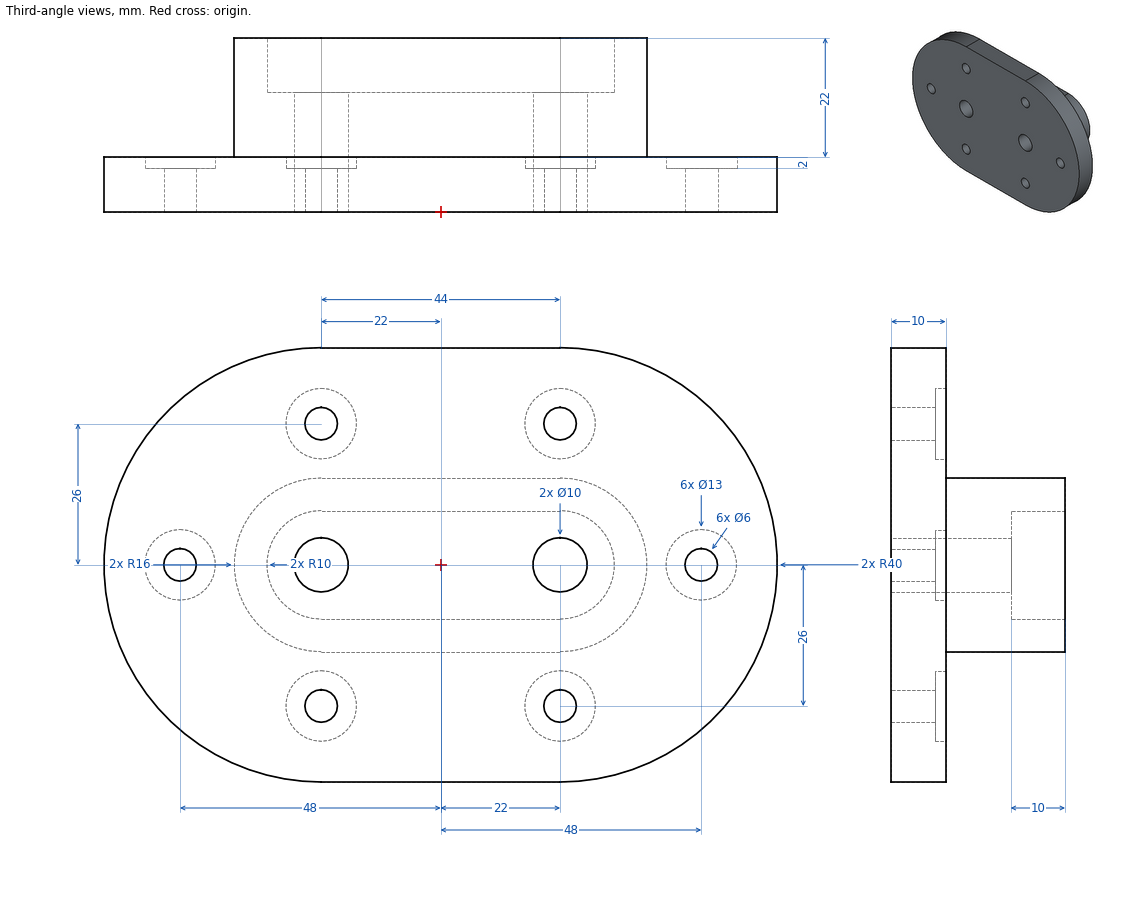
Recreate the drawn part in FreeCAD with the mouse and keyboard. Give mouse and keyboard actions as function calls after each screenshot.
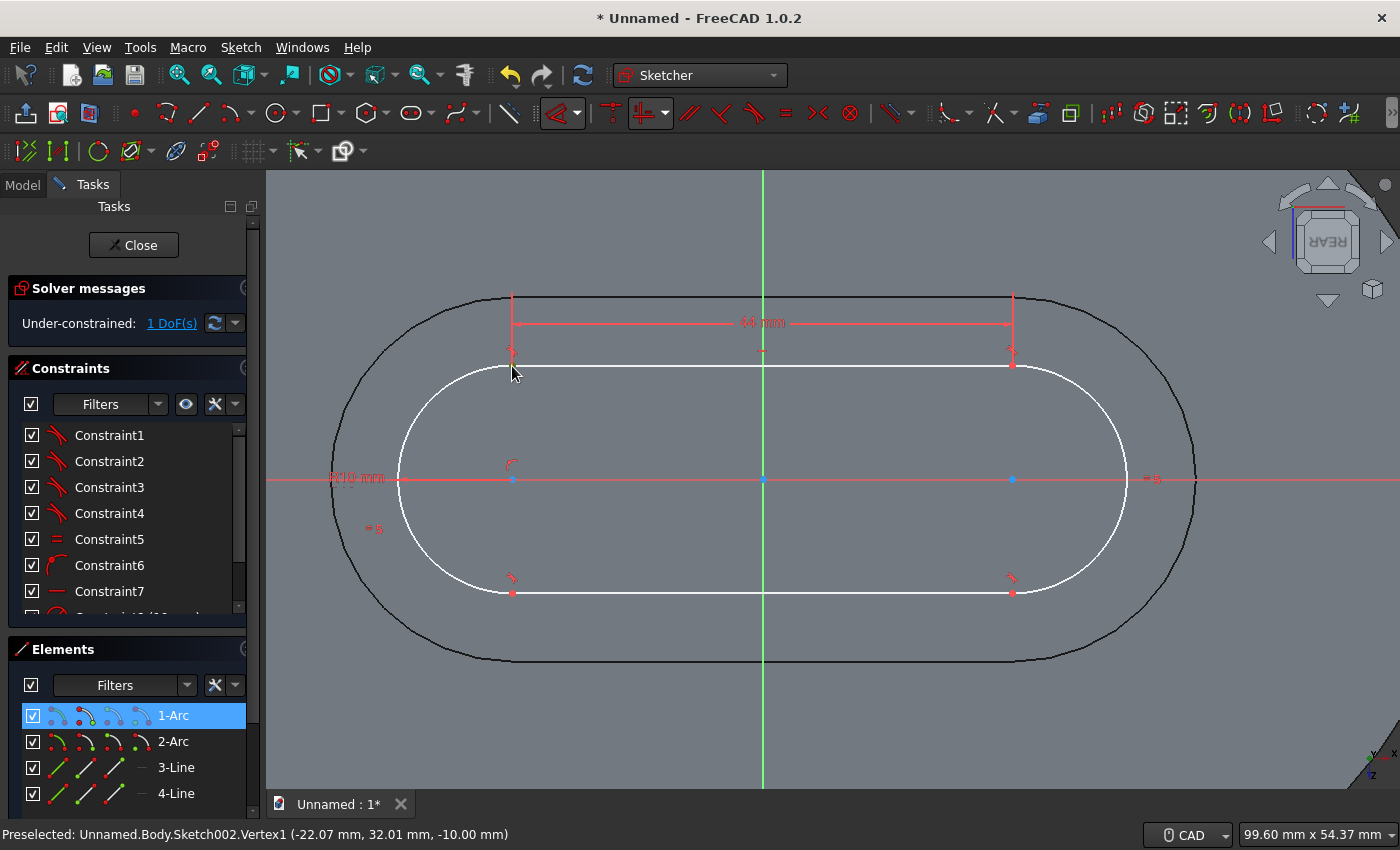
key(l)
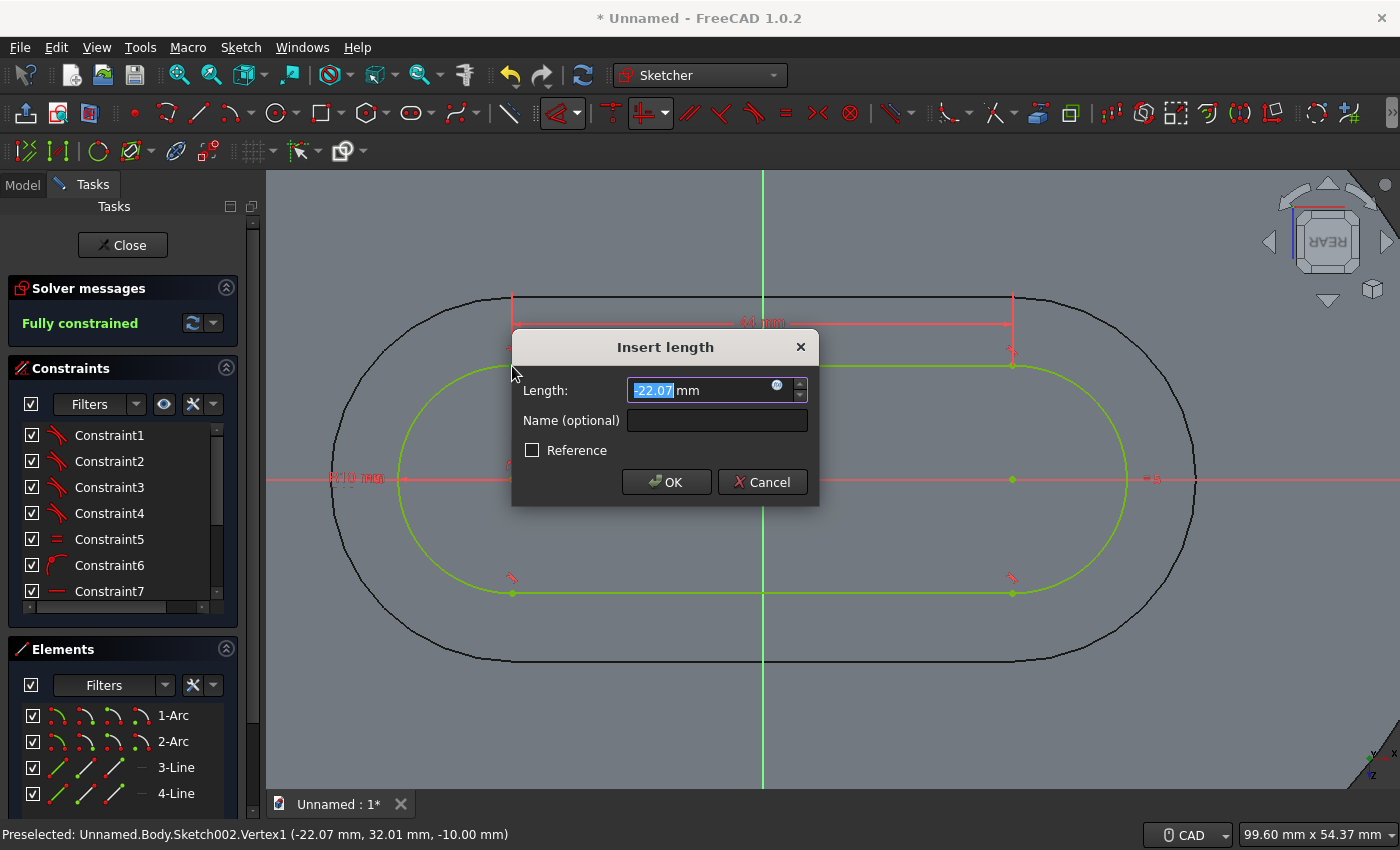
text(-22)
key(Return)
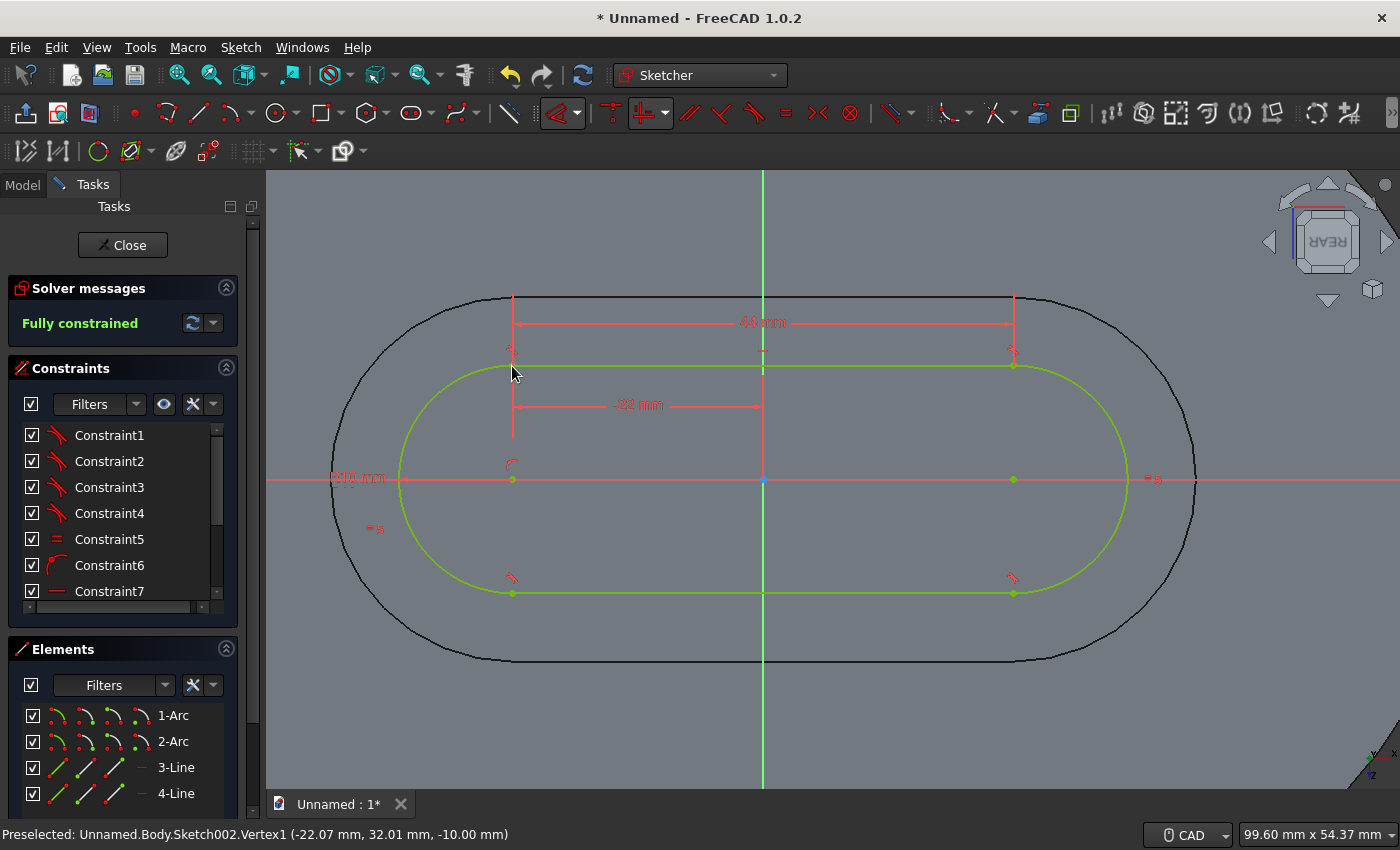
click(123, 245)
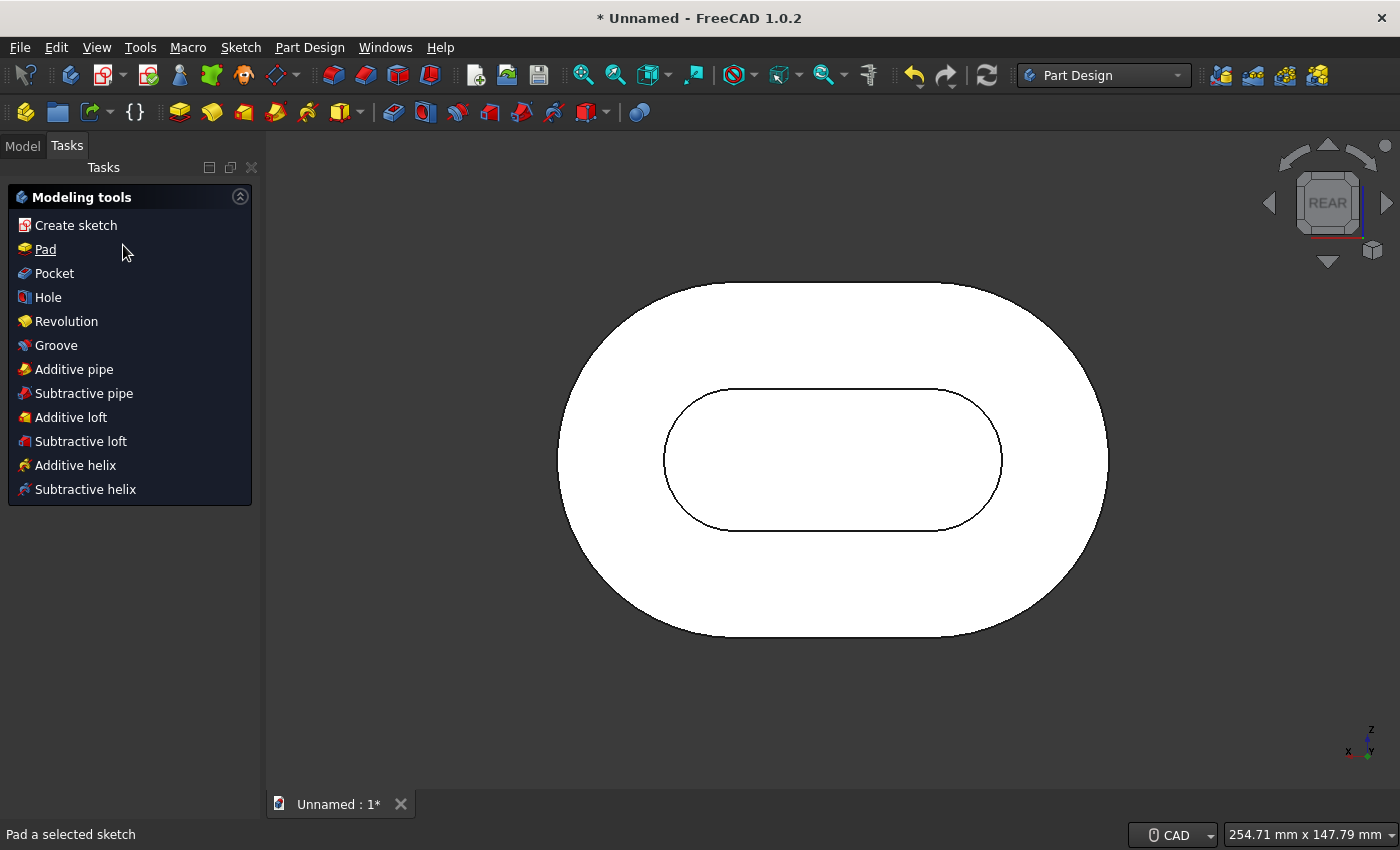
click(394, 112)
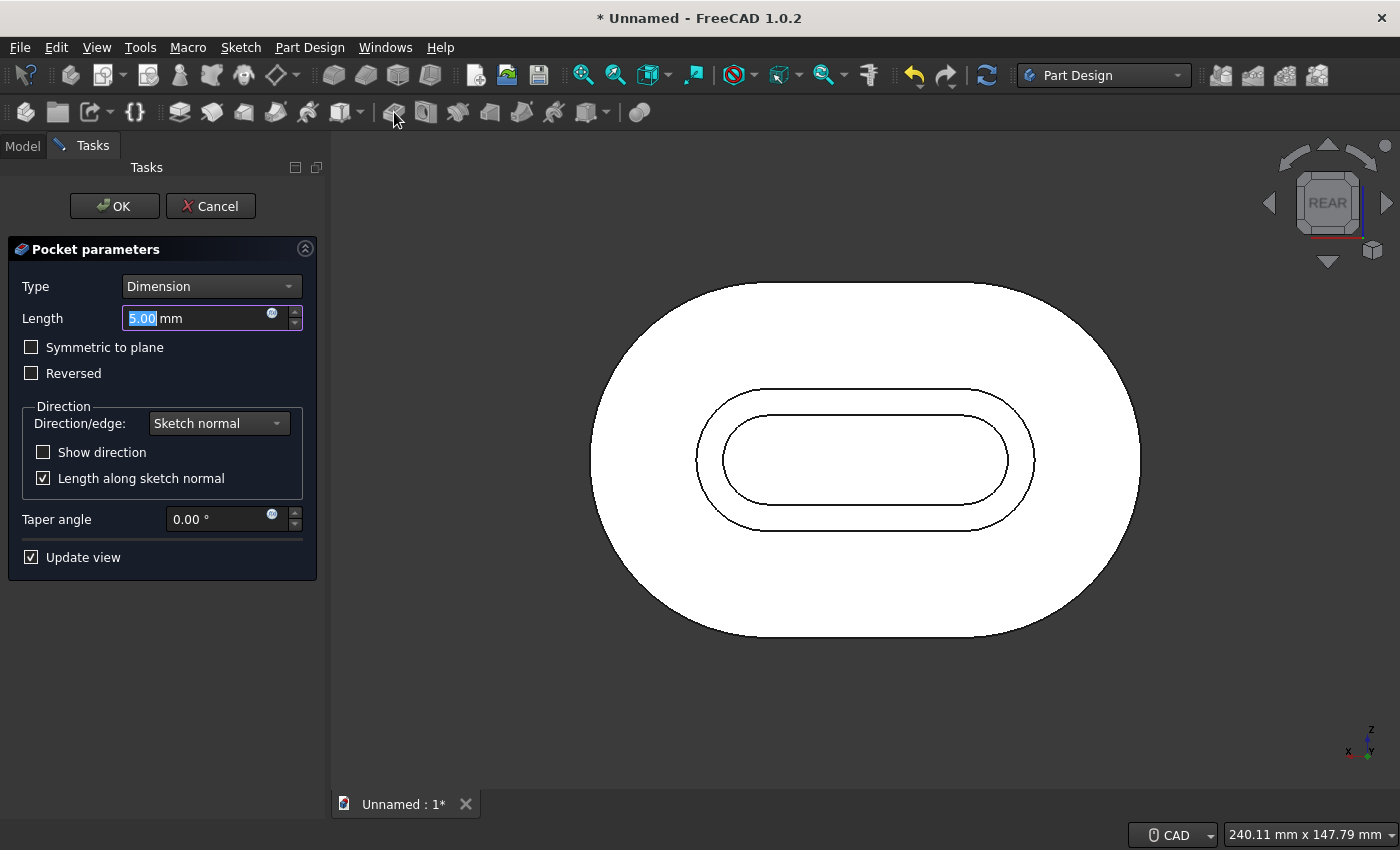
text(10)
key(Tab)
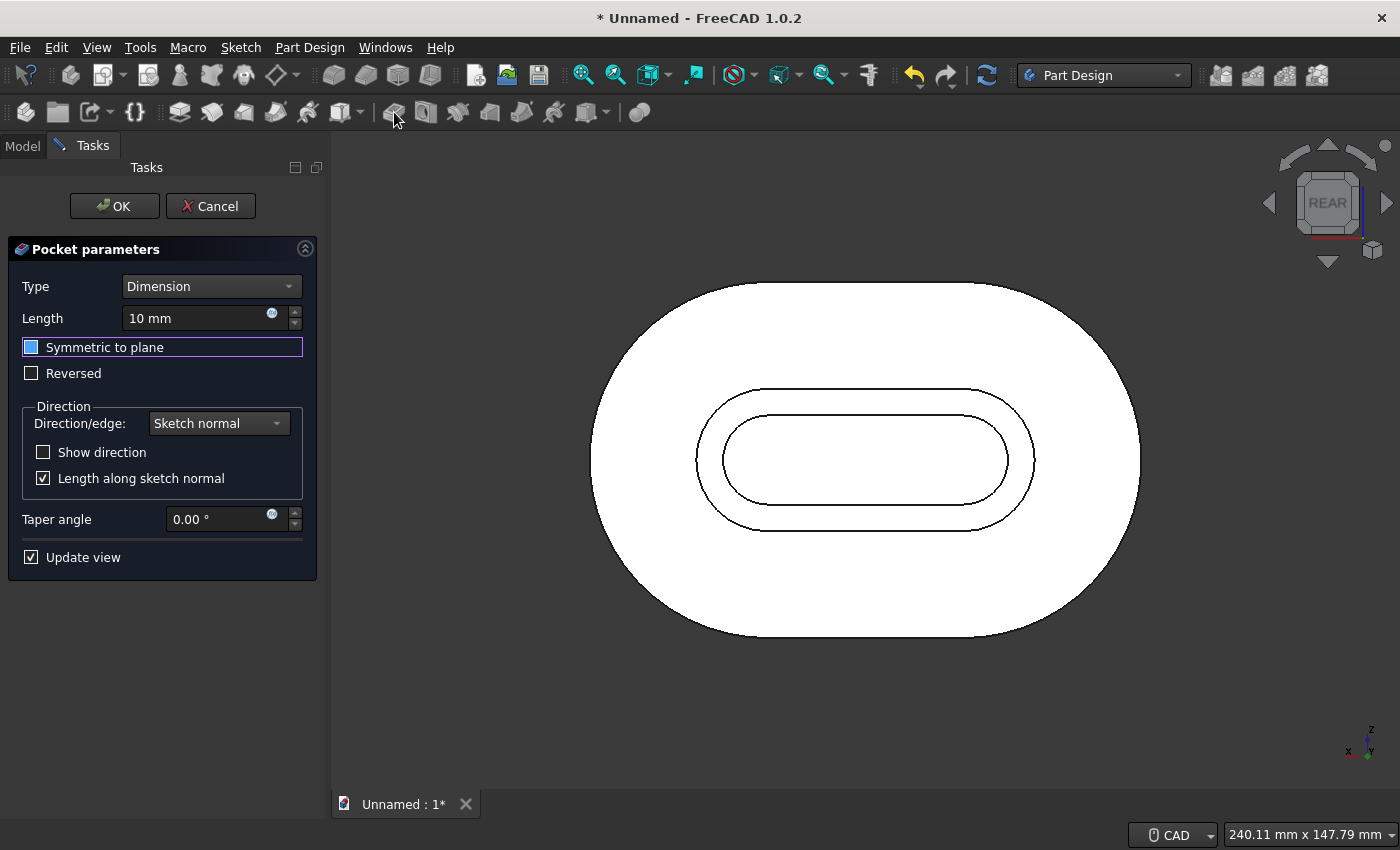
click(115, 206)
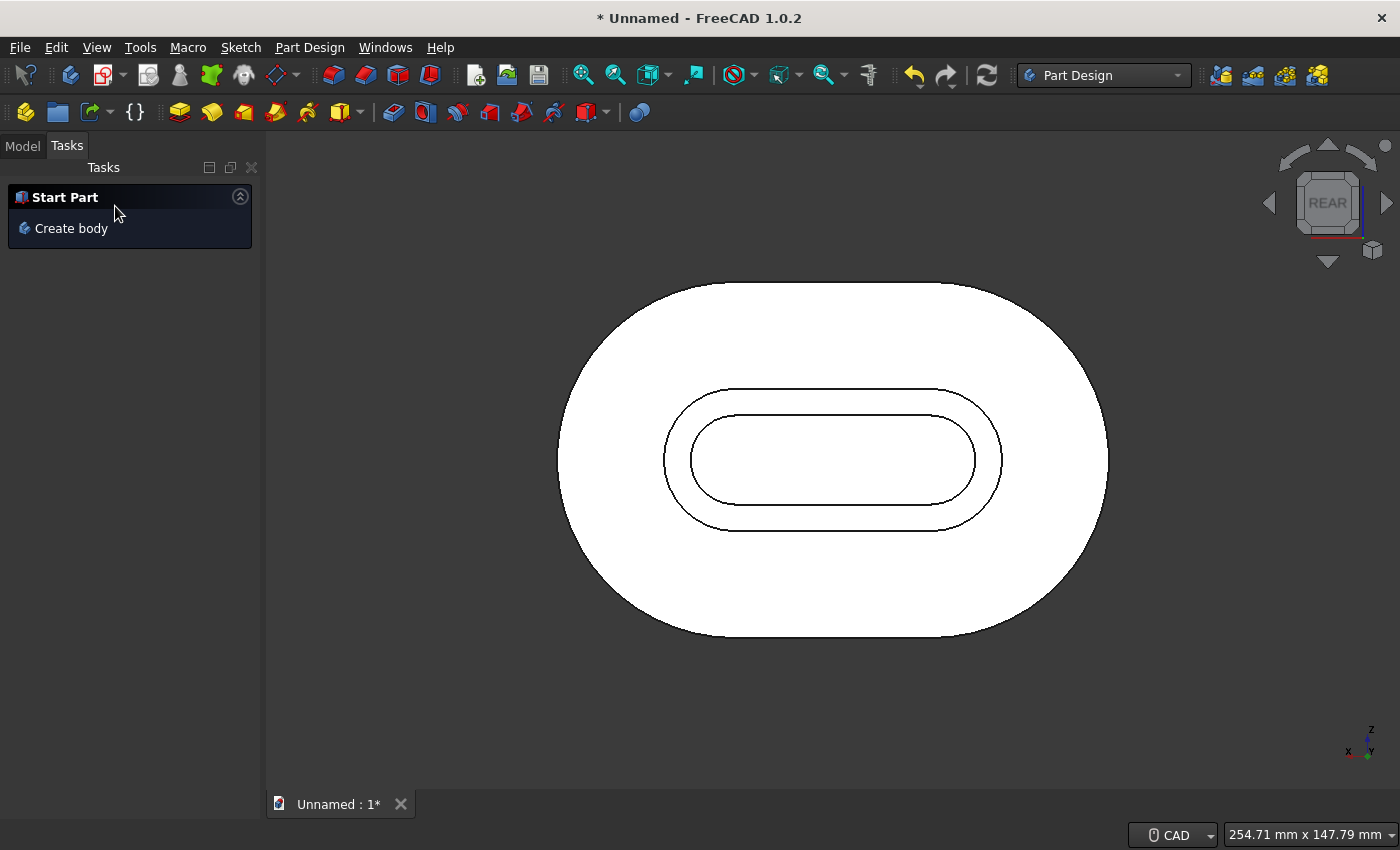
click(752, 459)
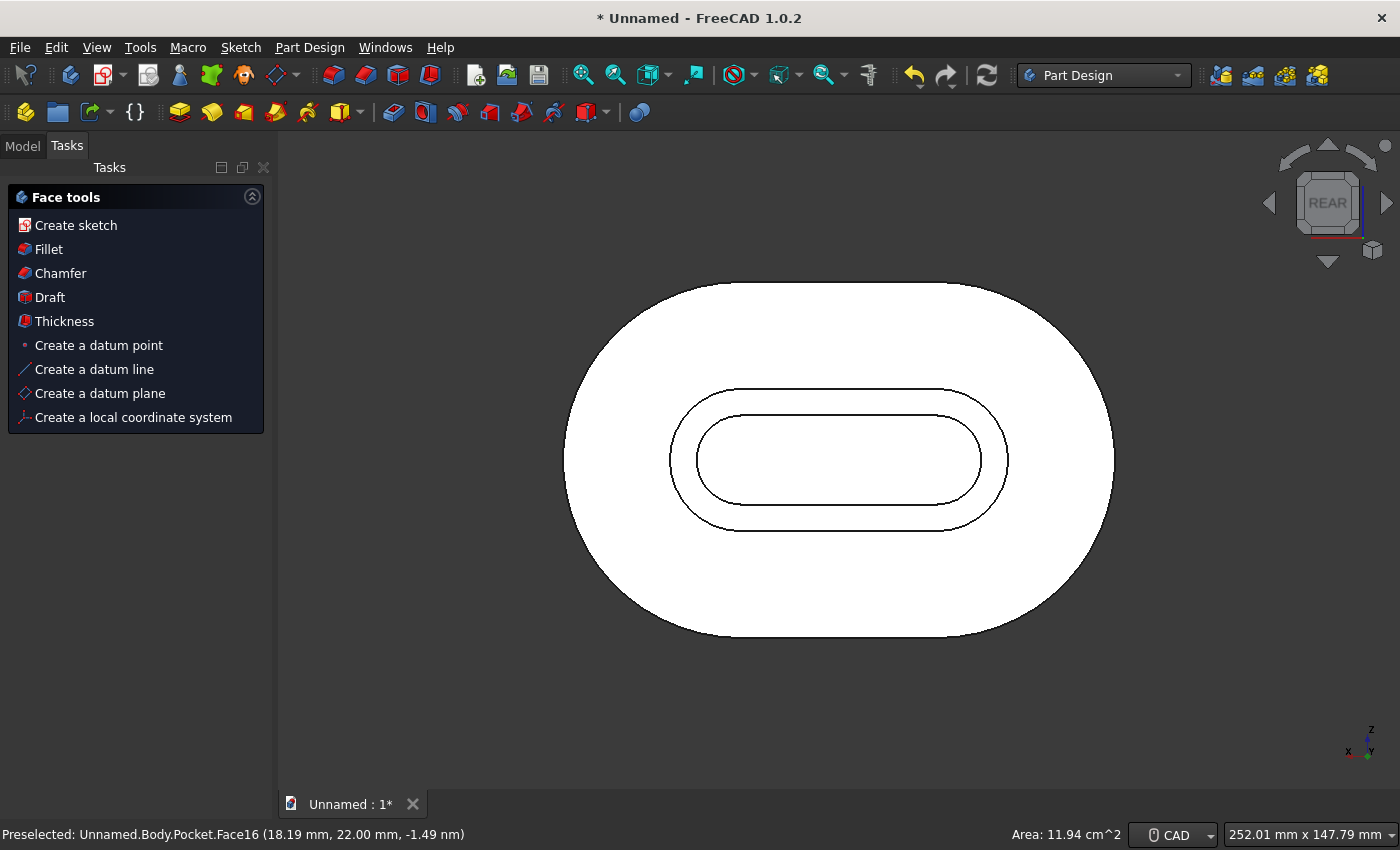
click(104, 76)